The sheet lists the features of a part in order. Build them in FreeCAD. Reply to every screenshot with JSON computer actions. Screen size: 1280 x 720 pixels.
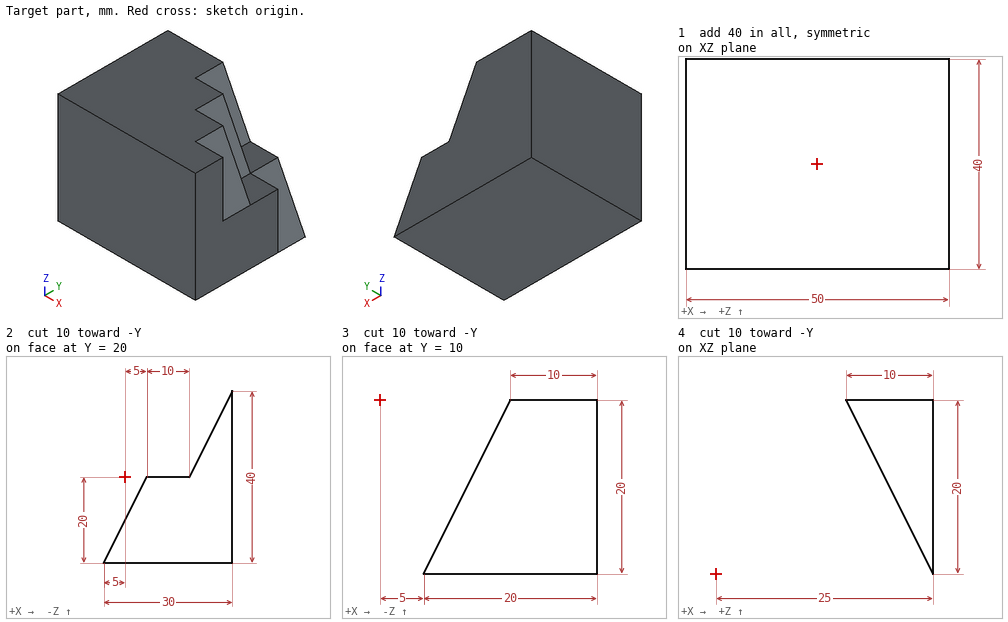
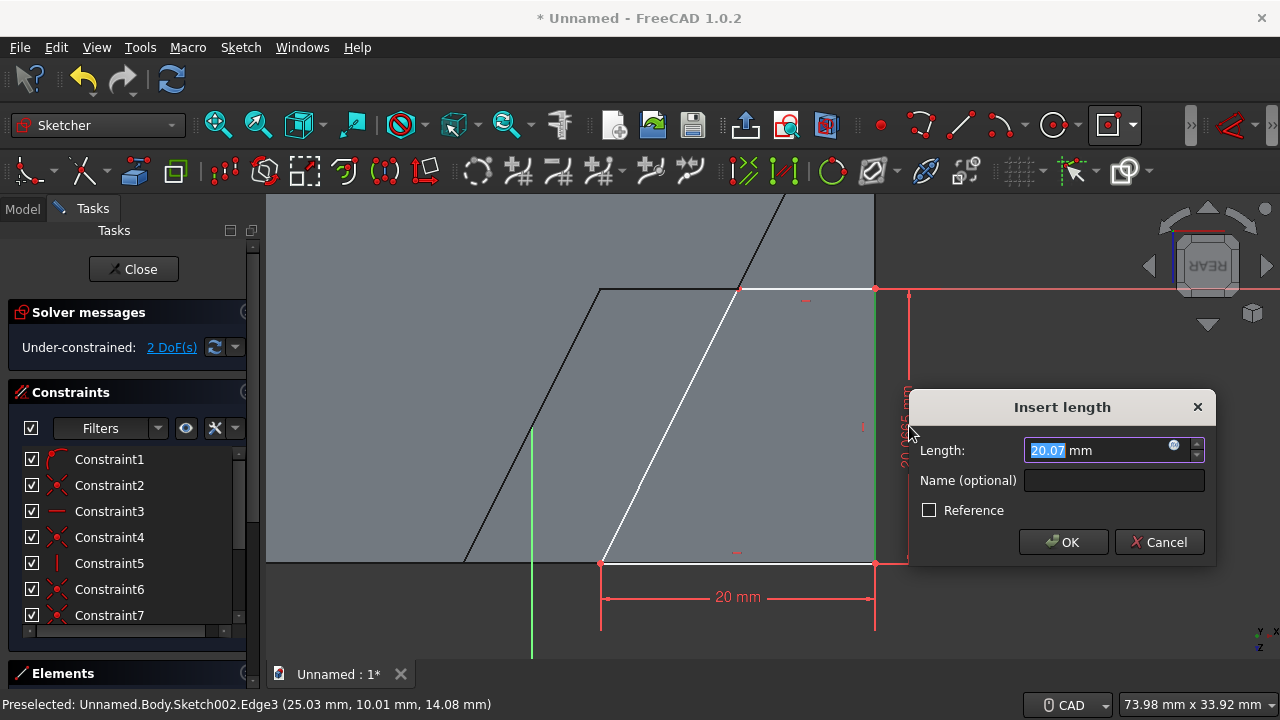
{"action": "type", "text": "20"}
{"action": "key", "text": "Return"}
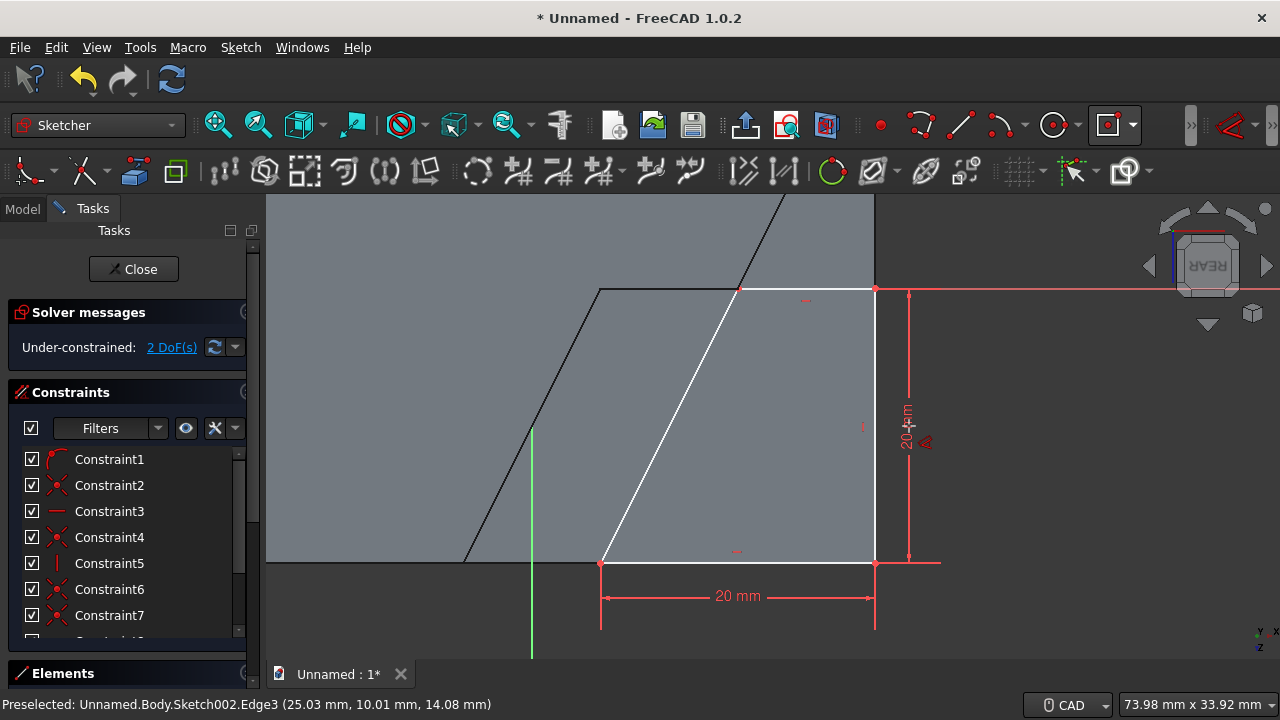
{"action": "left_click", "coordinate": [834, 289]}
{"action": "left_click", "coordinate": [807, 255]}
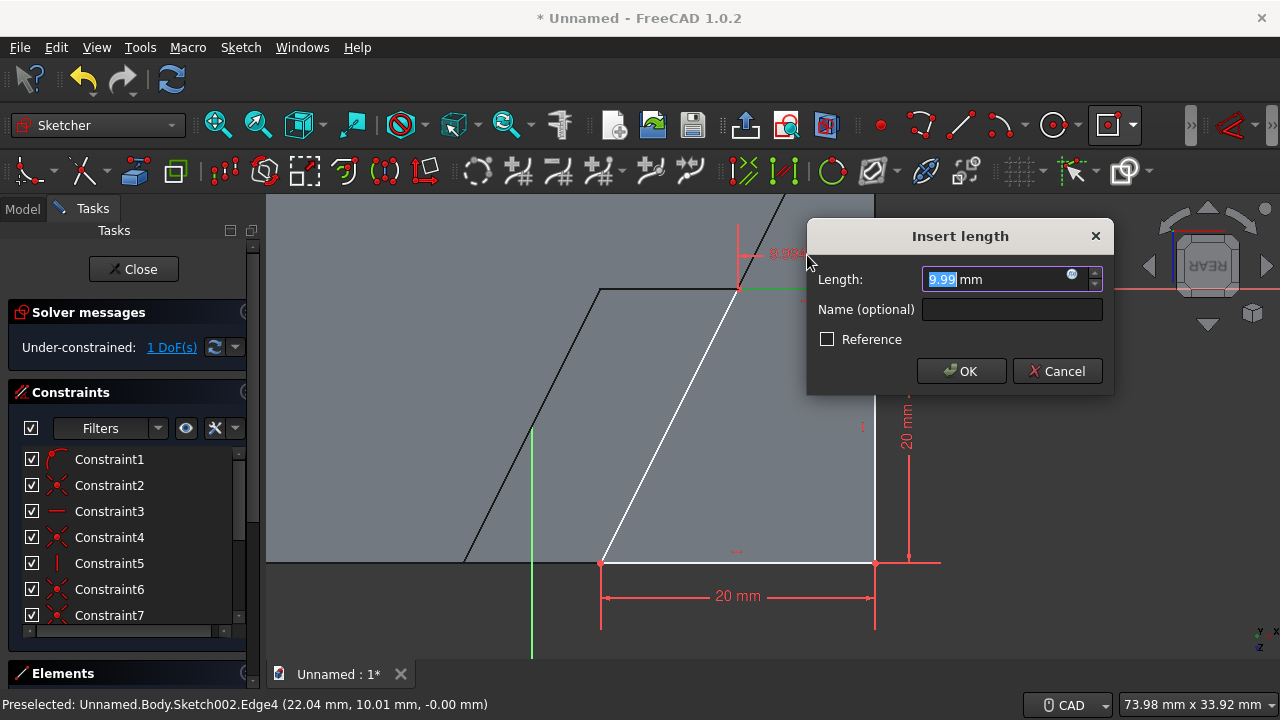
{"action": "type", "text": "10"}
{"action": "key", "text": "Return"}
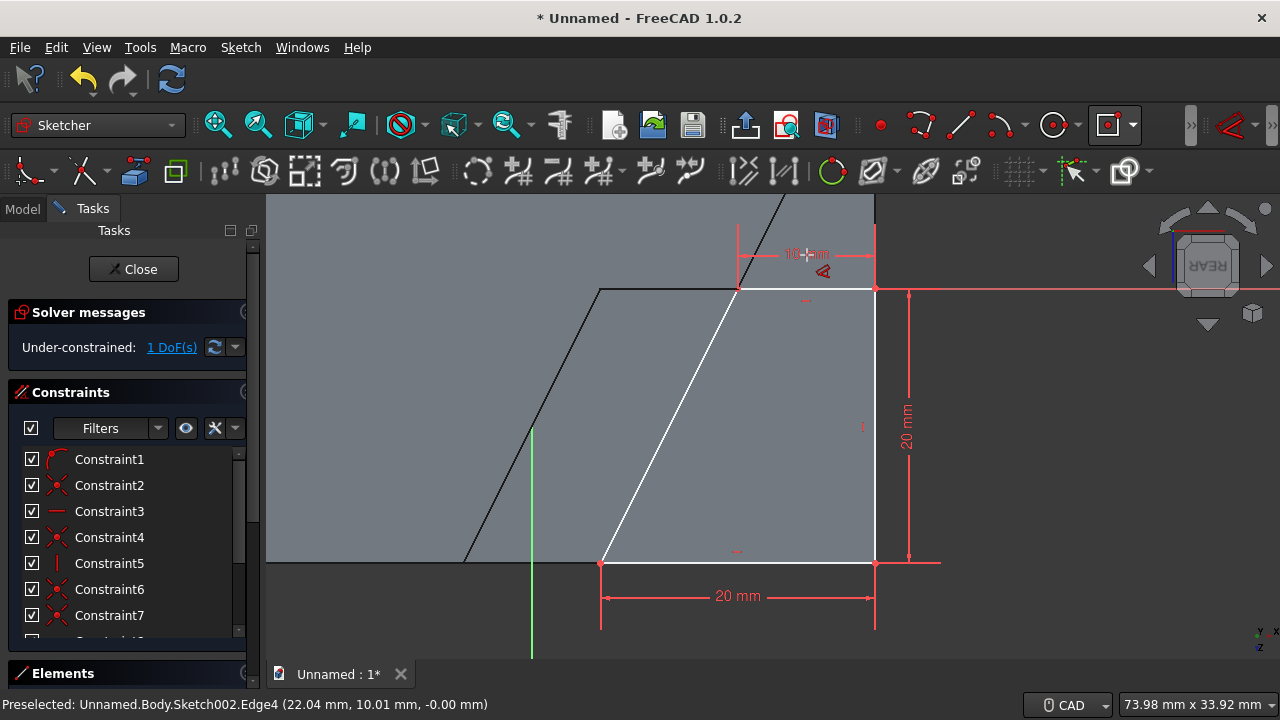
{"action": "left_click", "coordinate": [601, 563]}
{"action": "left_click", "coordinate": [566, 597]}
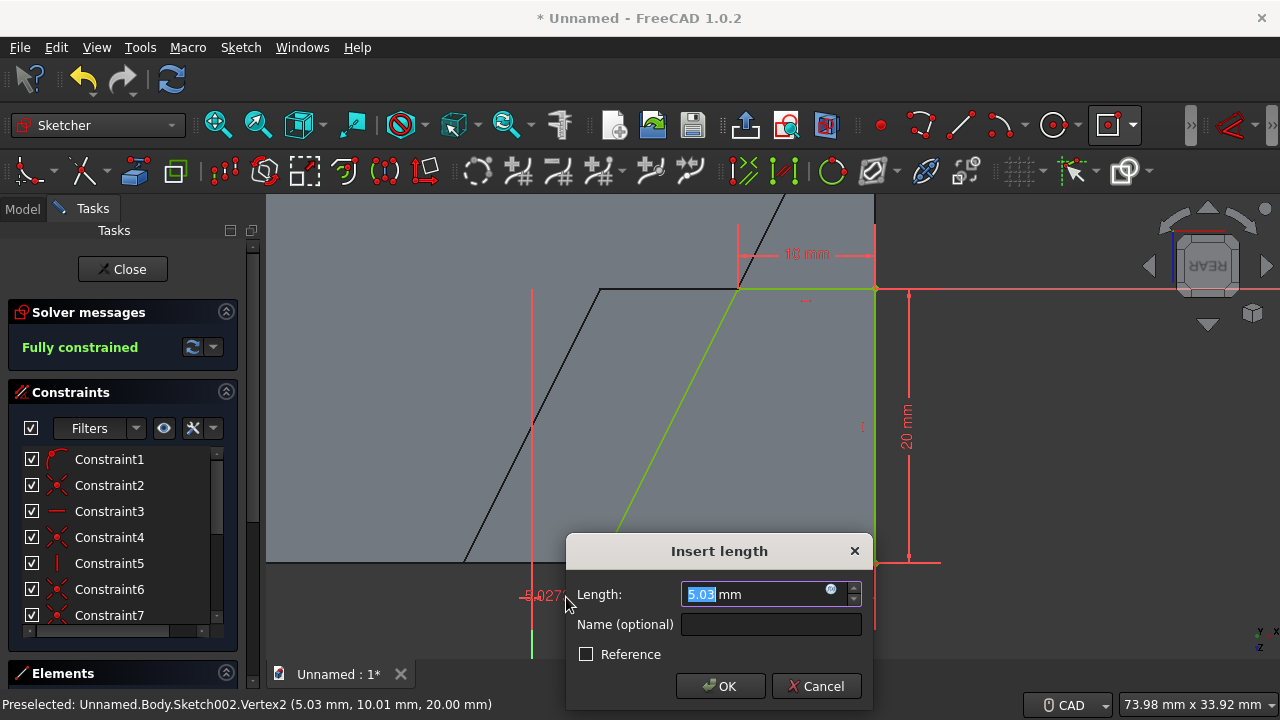
{"action": "type", "text": "5"}
{"action": "key", "text": "Return"}
{"action": "key", "text": "Escape"}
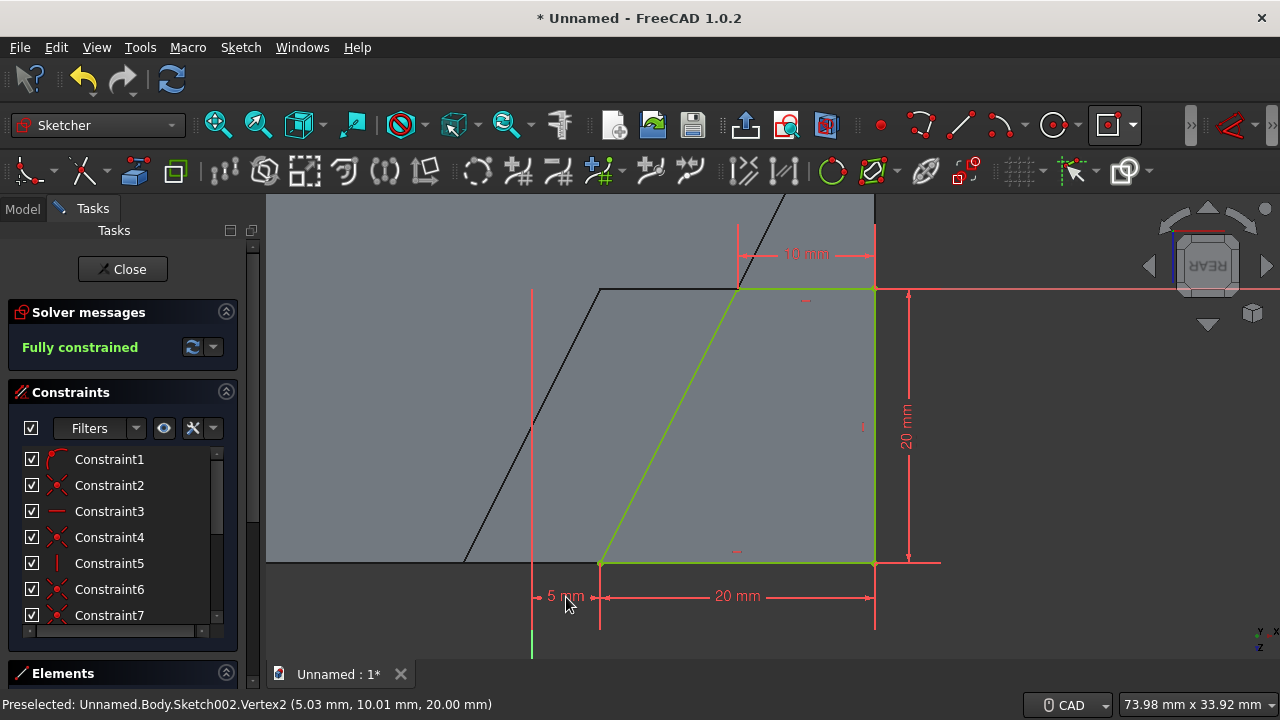
{"action": "left_click", "coordinate": [123, 269]}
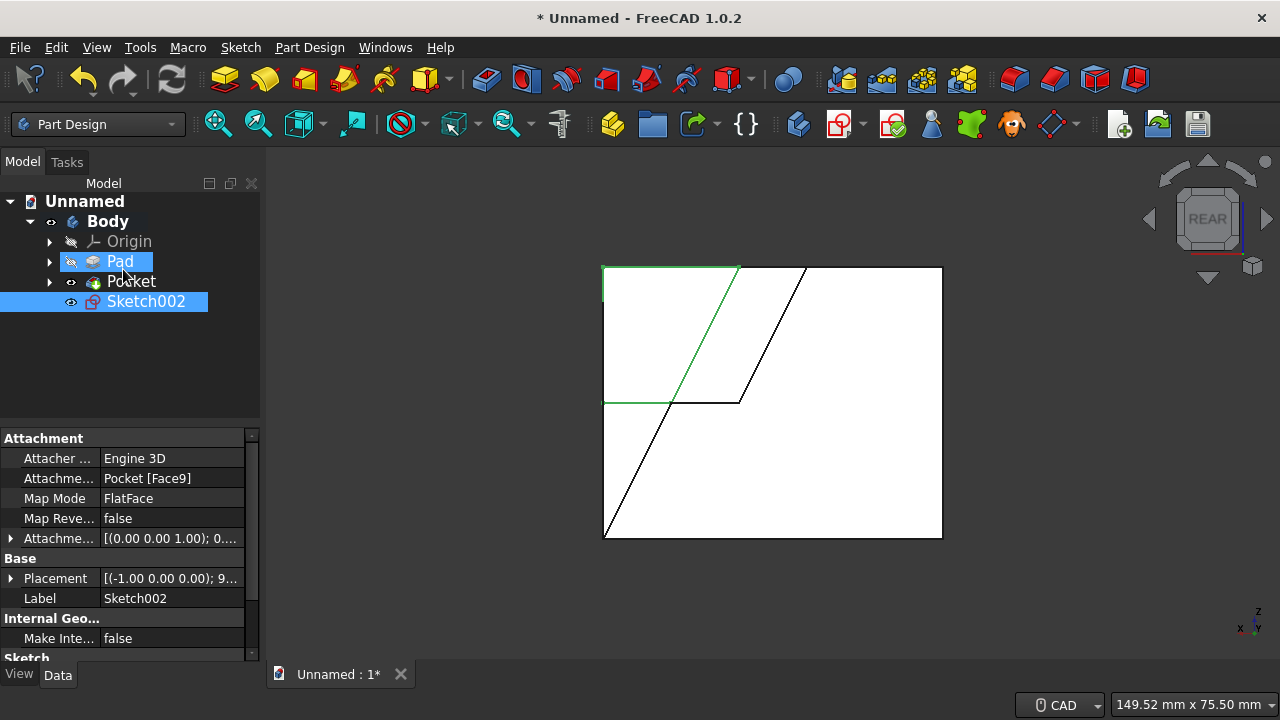
{"action": "left_click", "coordinate": [488, 80]}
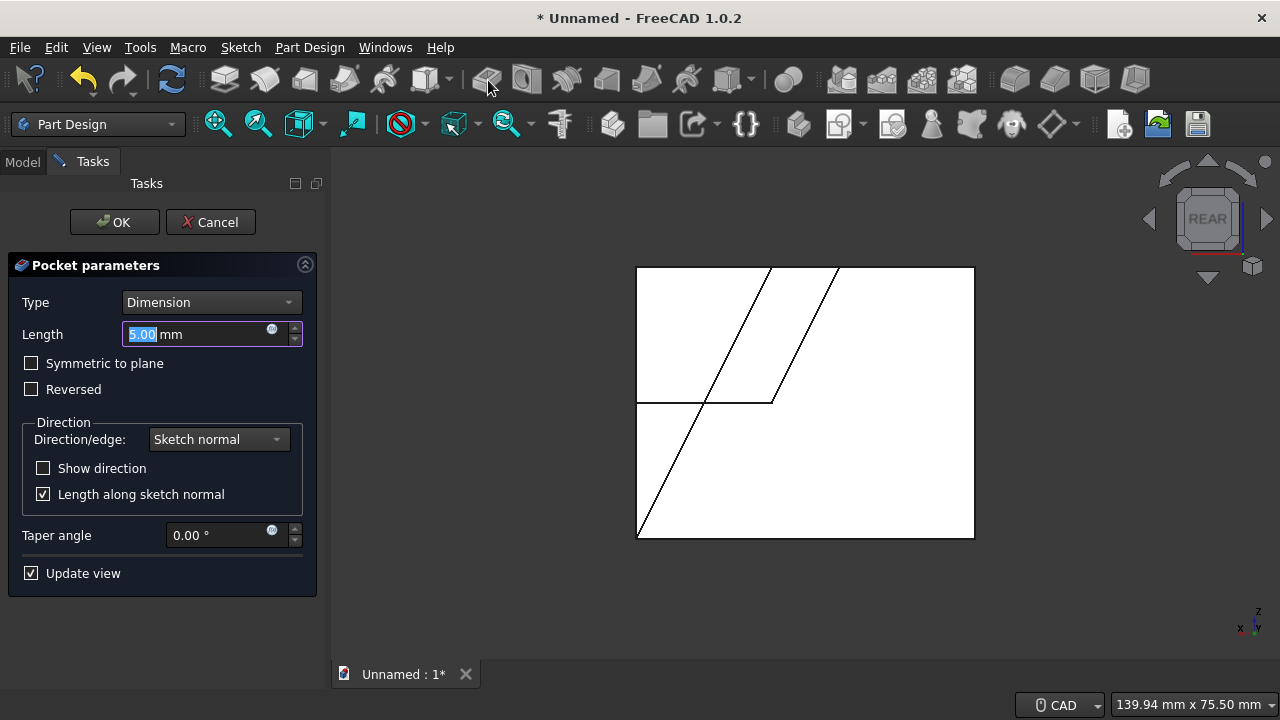
{"action": "type", "text": "10"}
{"action": "key", "text": "Tab"}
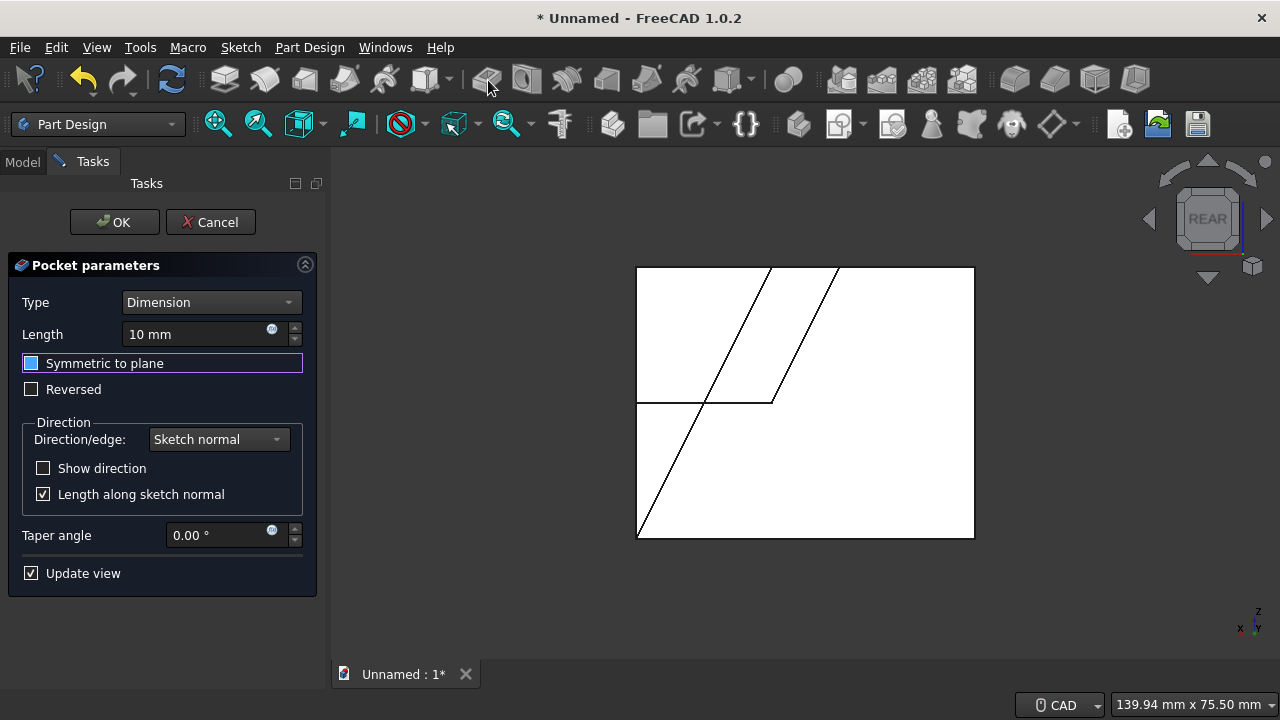
{"action": "left_click", "coordinate": [115, 222]}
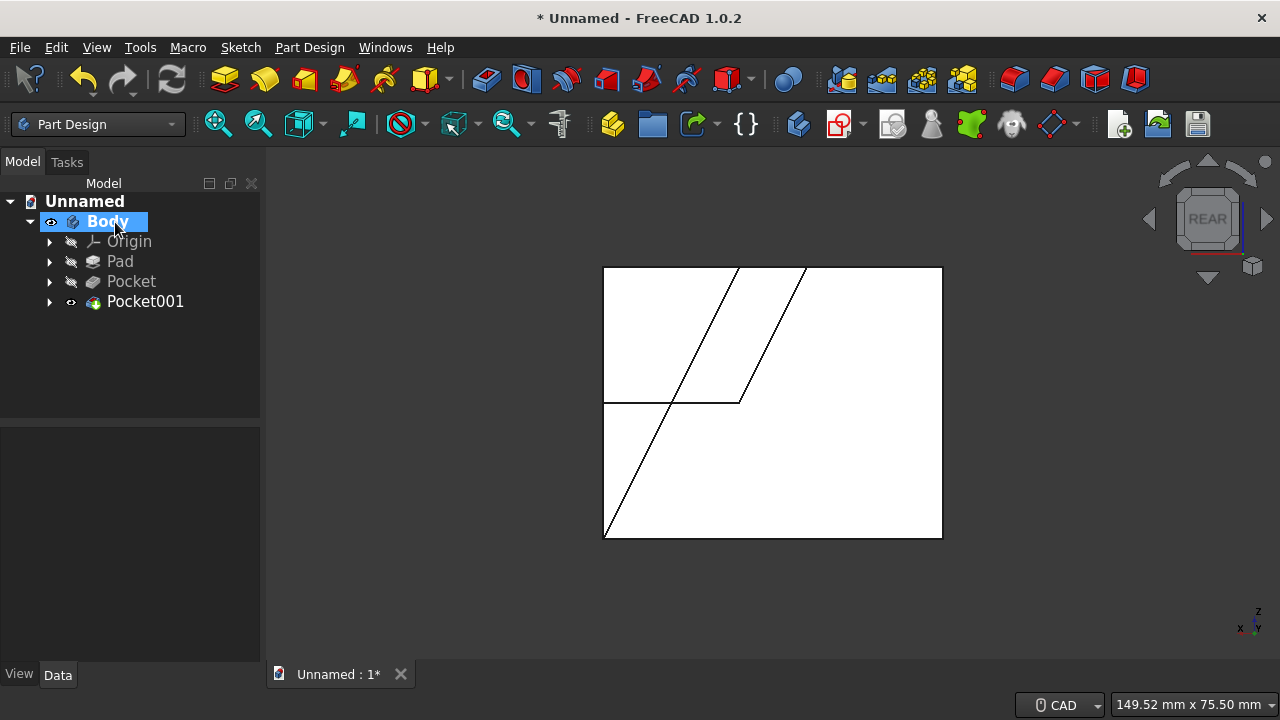
{"action": "left_click", "coordinate": [840, 124]}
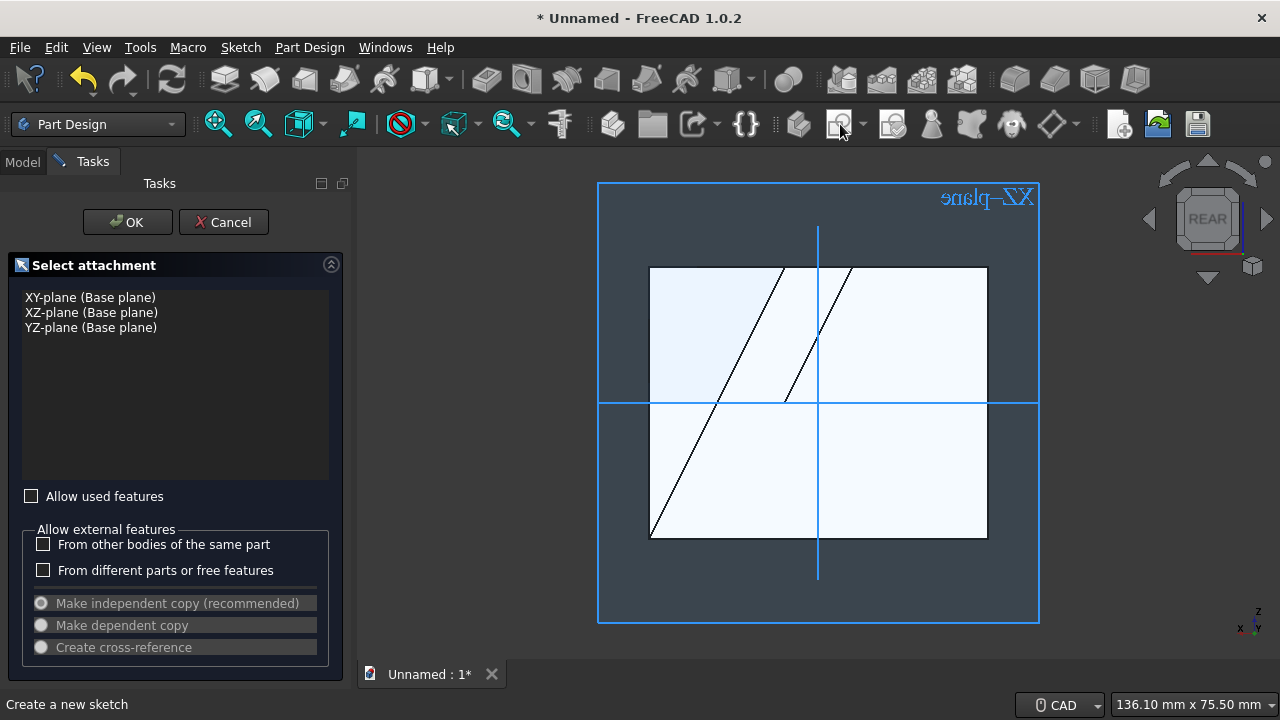
{"action": "left_click", "coordinate": [82, 312]}